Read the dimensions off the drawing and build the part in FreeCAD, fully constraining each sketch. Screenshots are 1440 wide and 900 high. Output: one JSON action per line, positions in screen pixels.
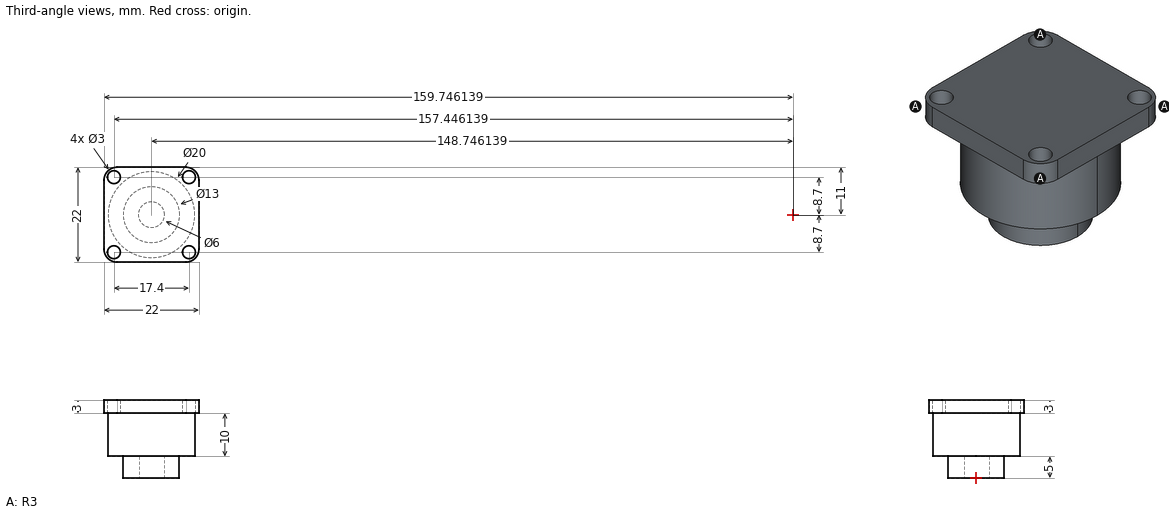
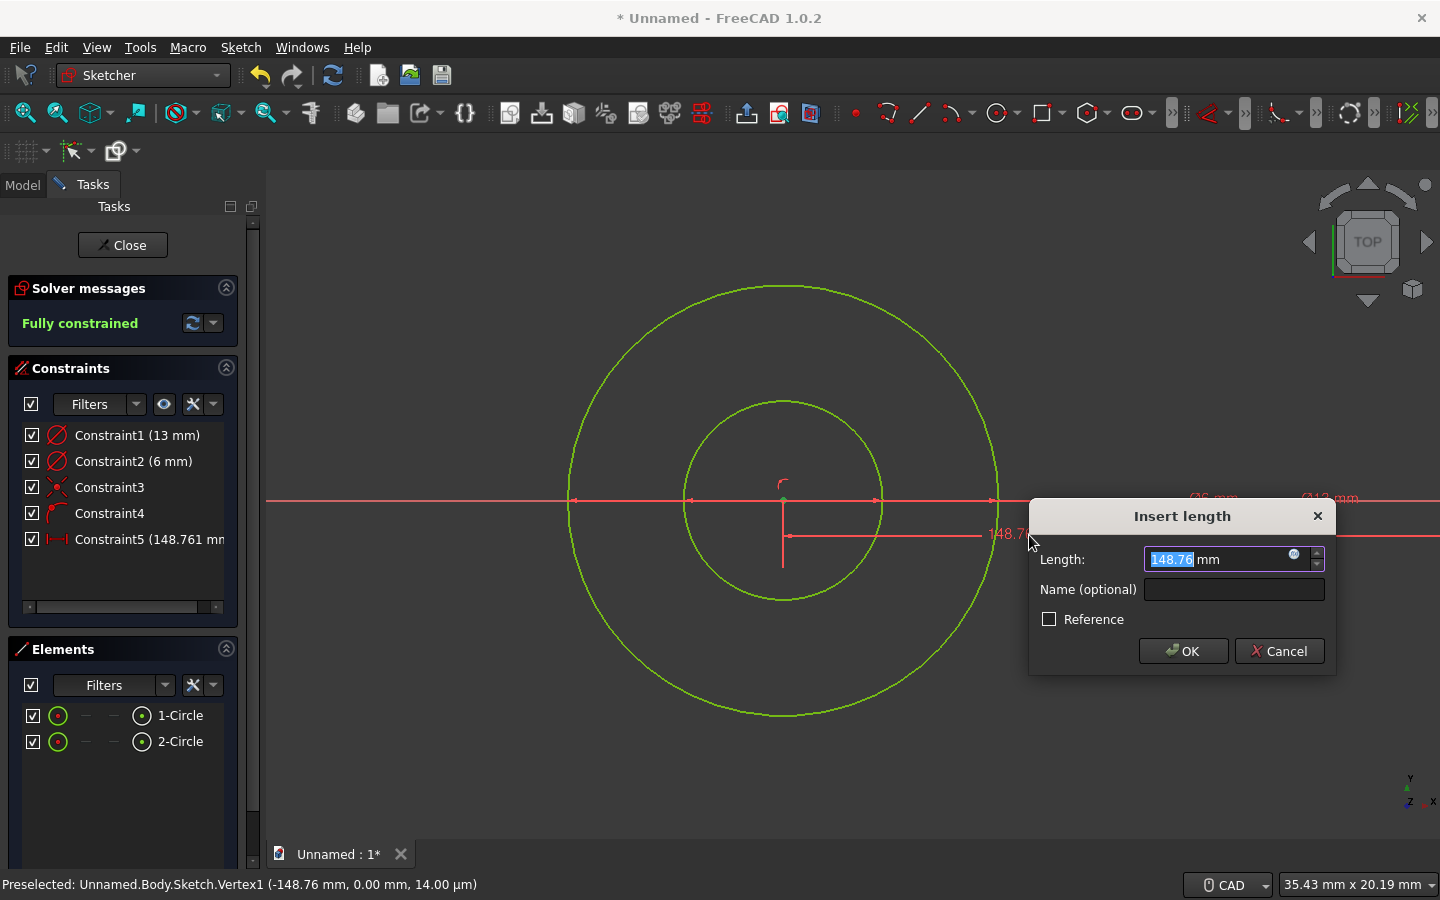
{"action": "type", "text": "148.746139"}
{"action": "key", "text": "Return"}
{"action": "key", "text": "Escape"}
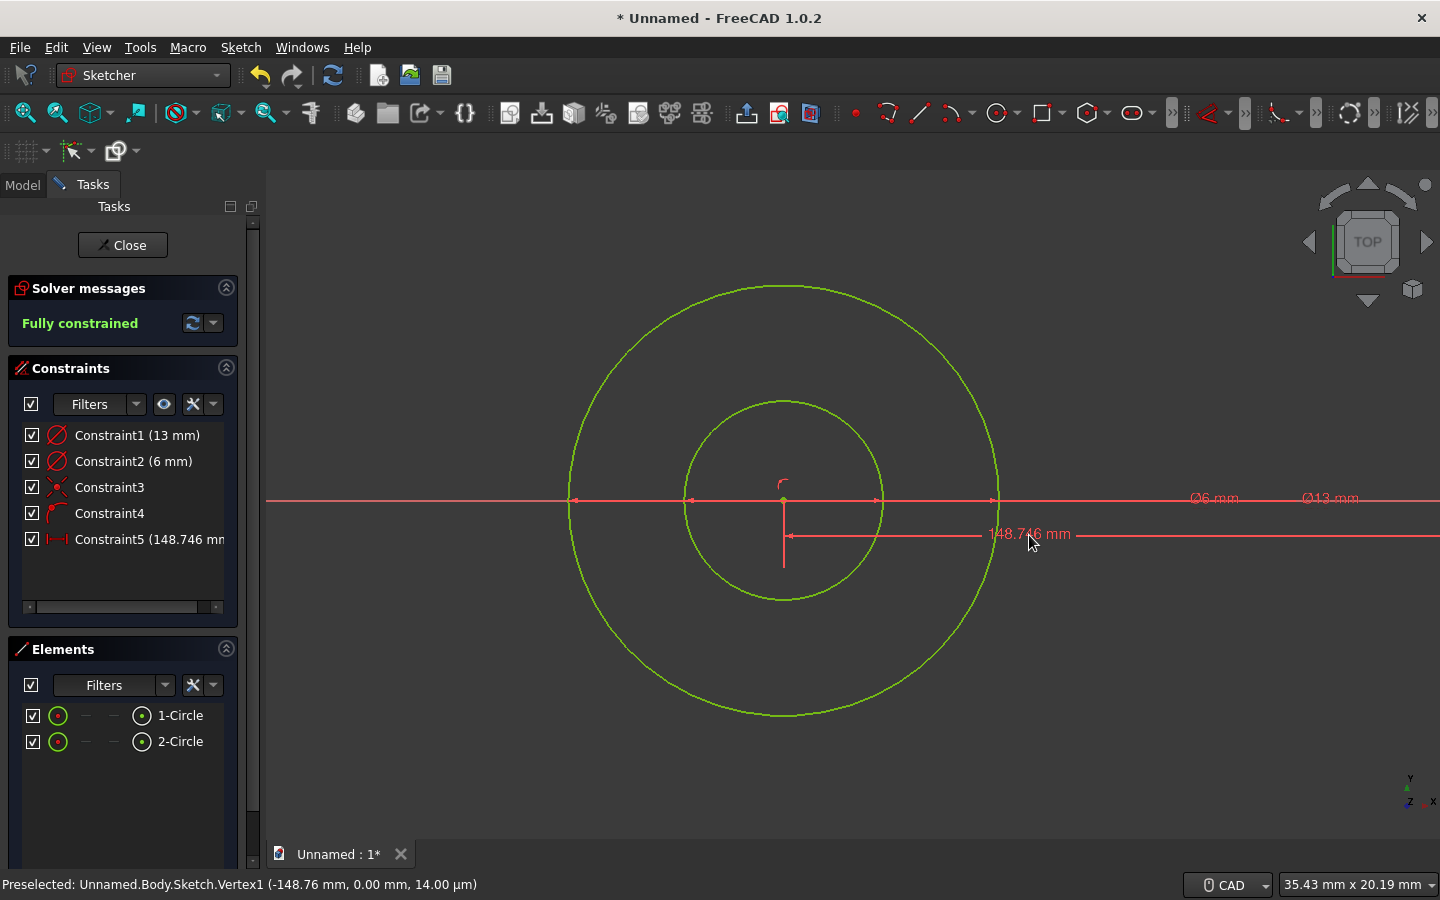
{"action": "left_click", "coordinate": [123, 245]}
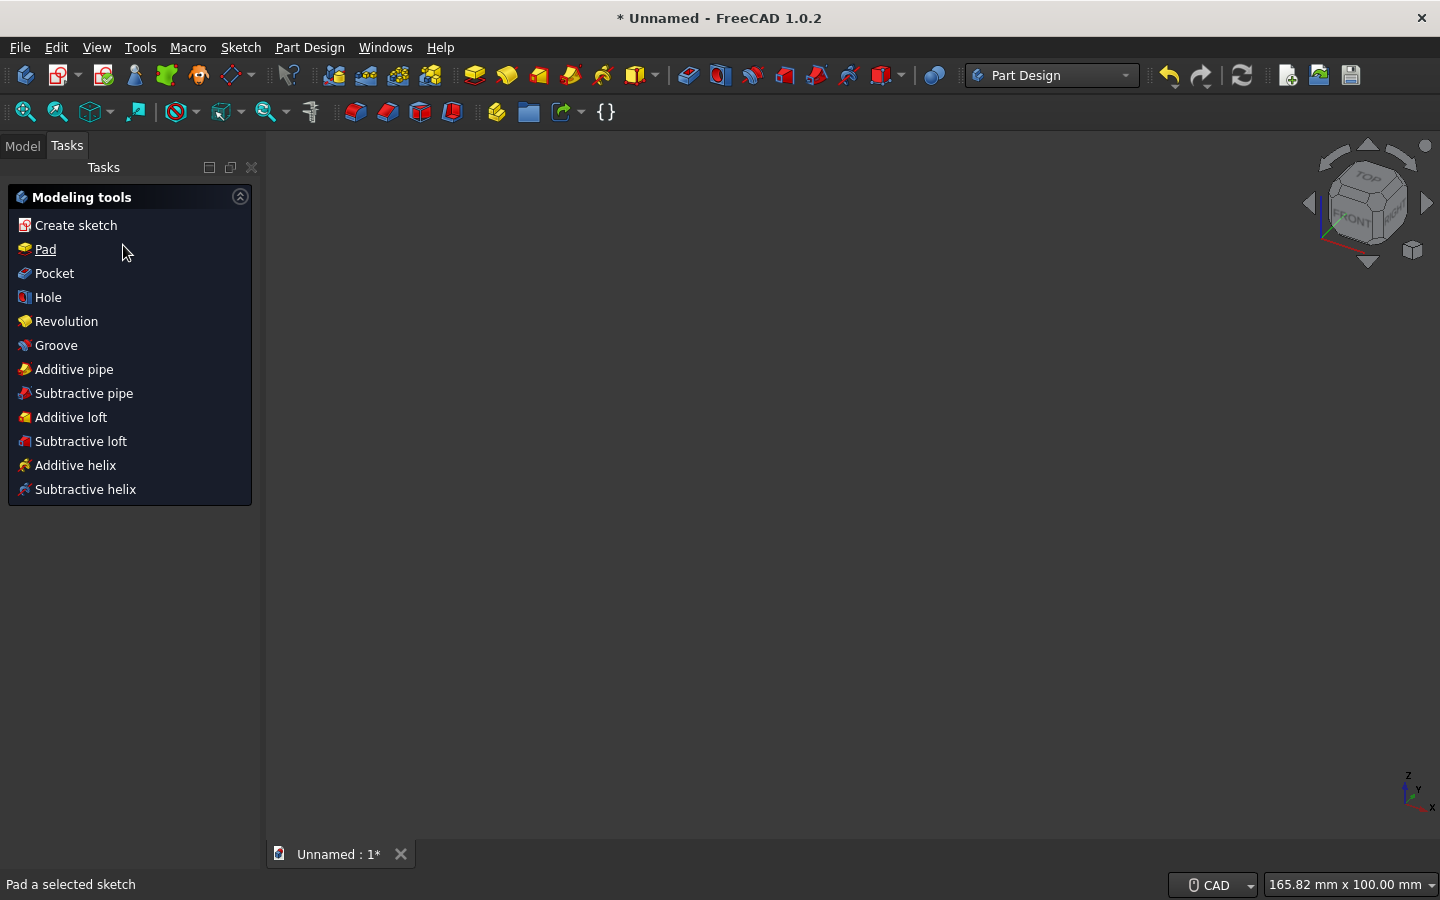
{"action": "left_click", "coordinate": [476, 76]}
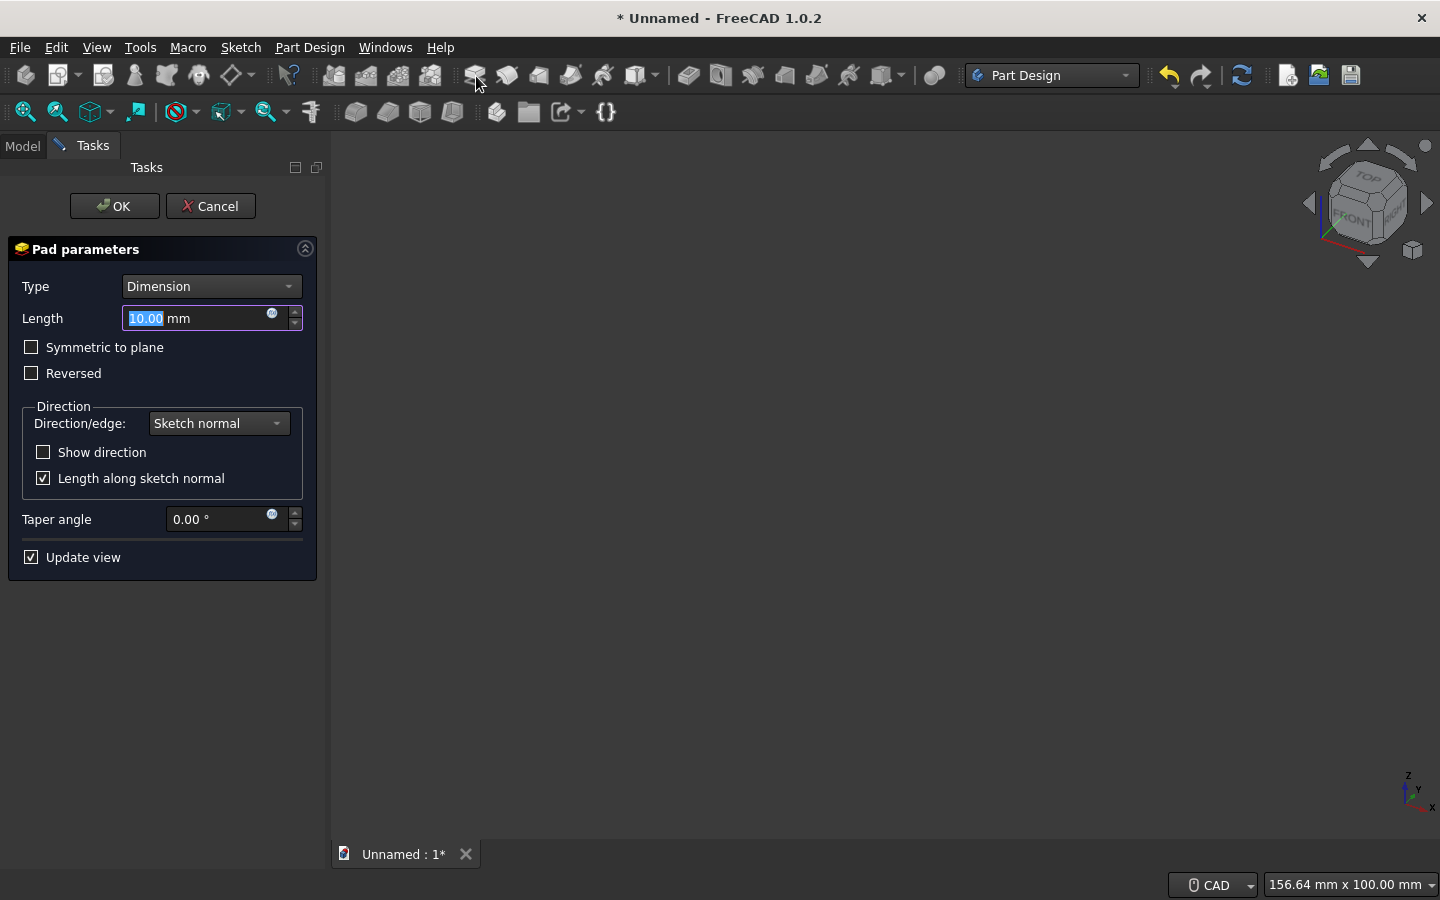
{"action": "type", "text": "5"}
{"action": "key", "text": "Tab"}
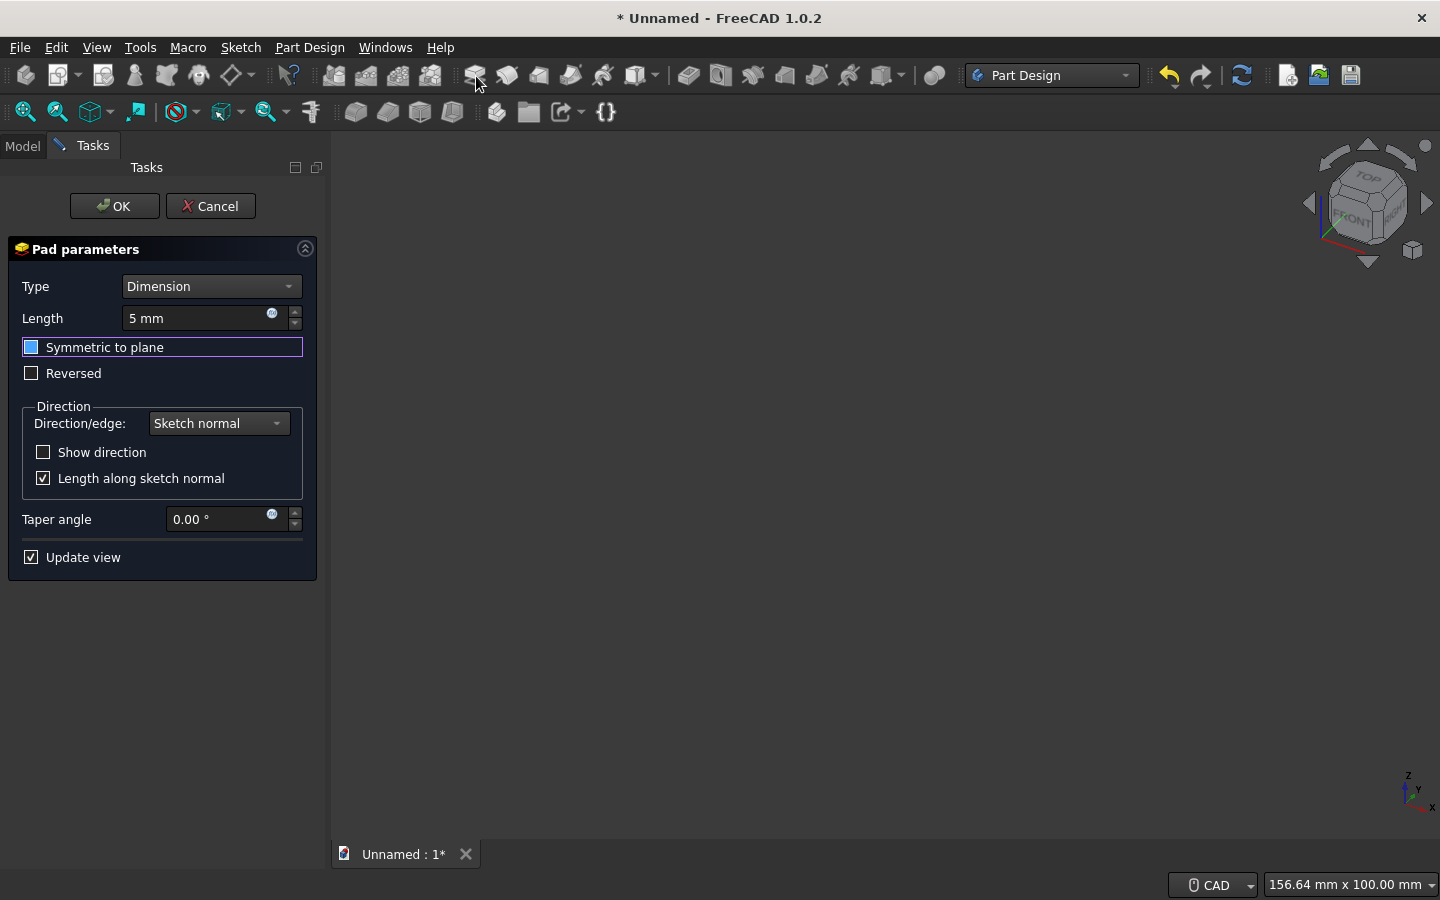
{"action": "left_click", "coordinate": [115, 206]}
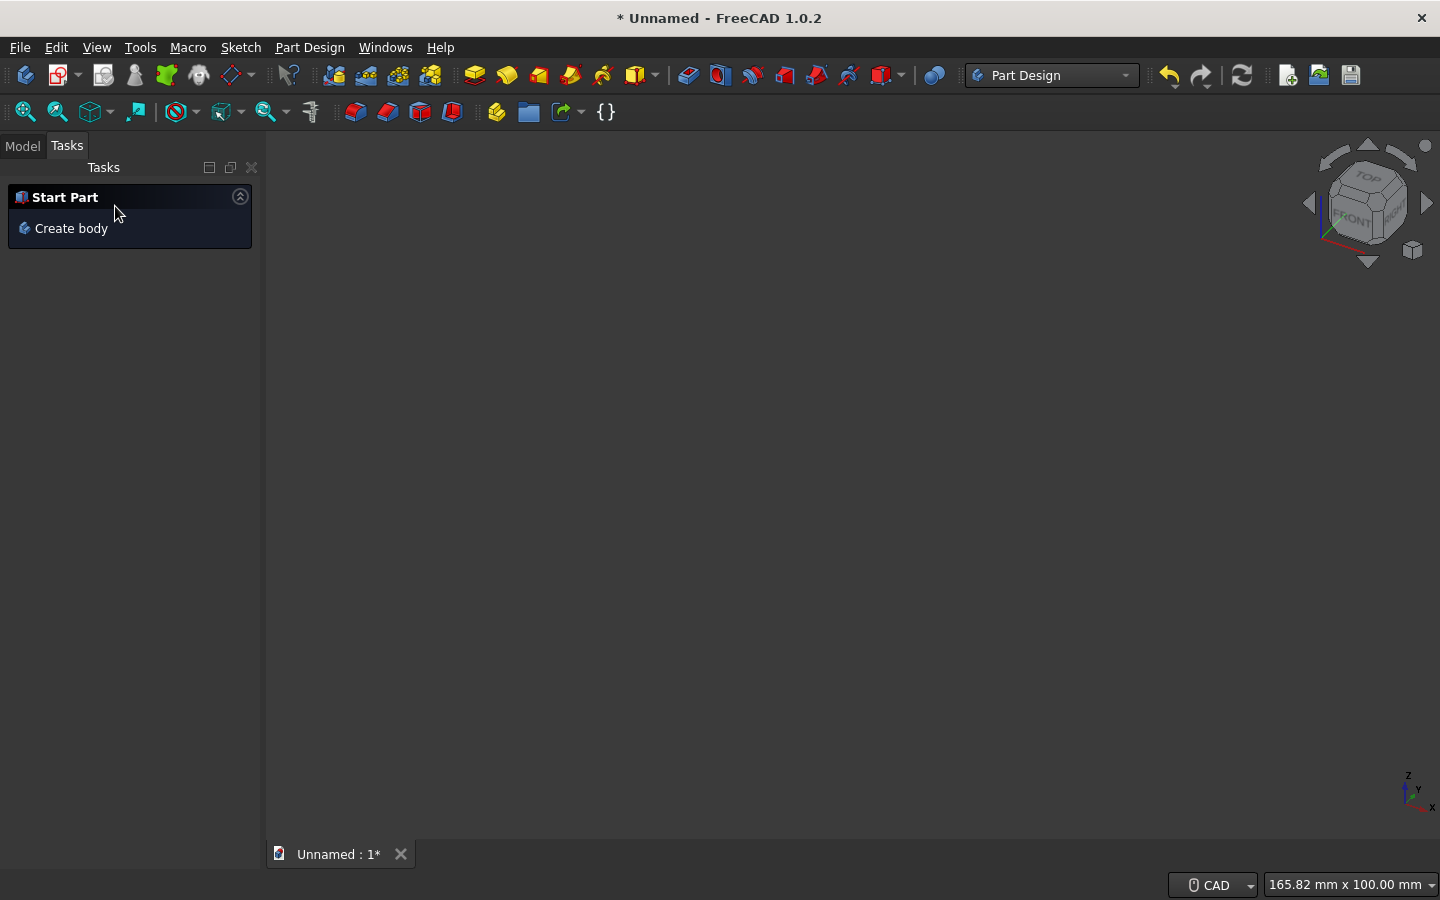
{"action": "left_click", "coordinate": [26, 112]}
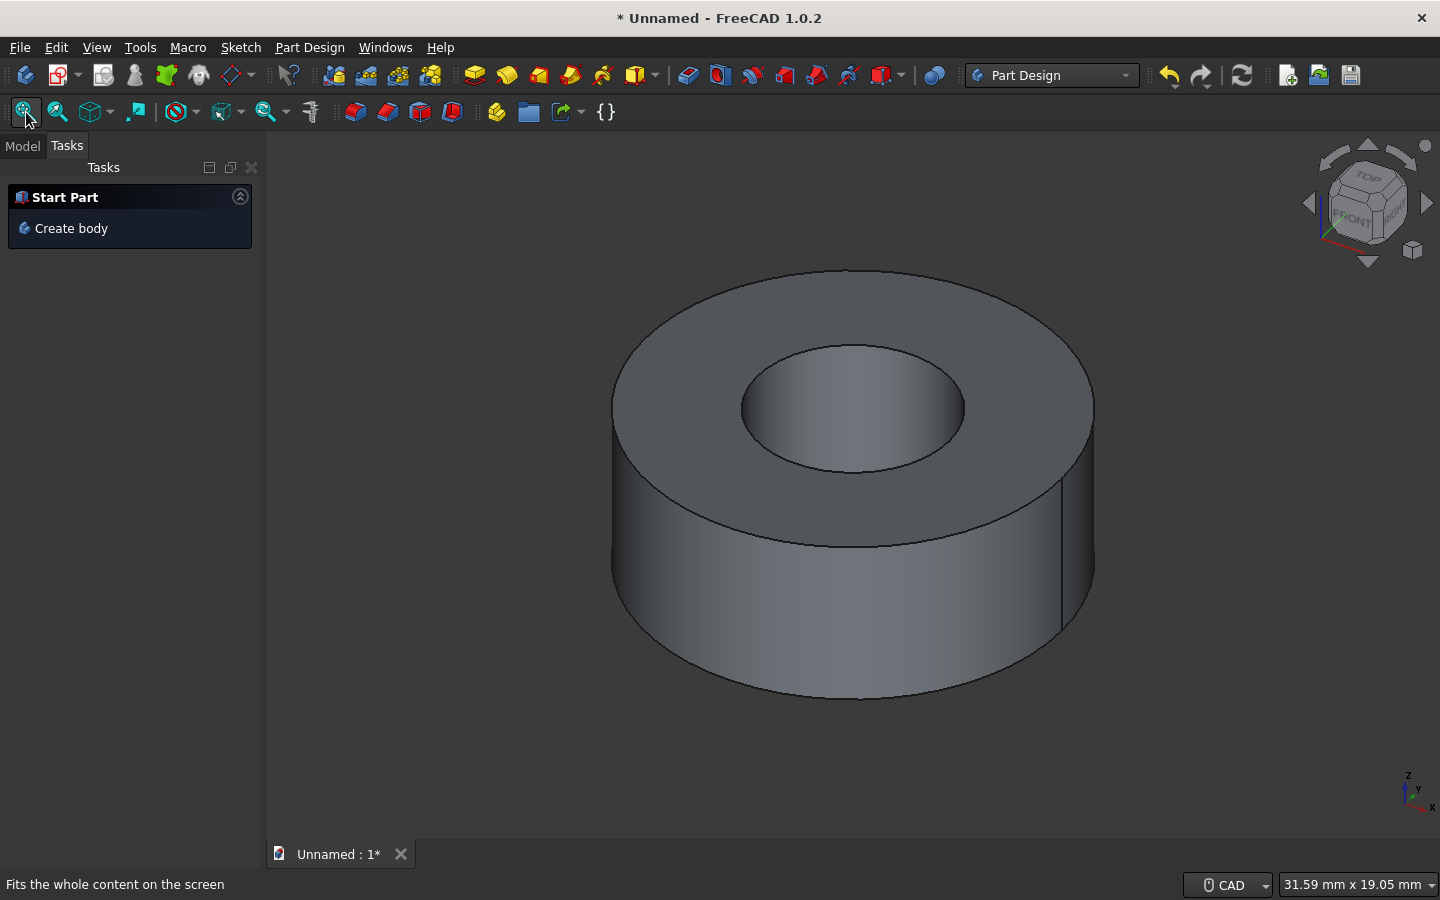
{"action": "left_click", "coordinate": [904, 516]}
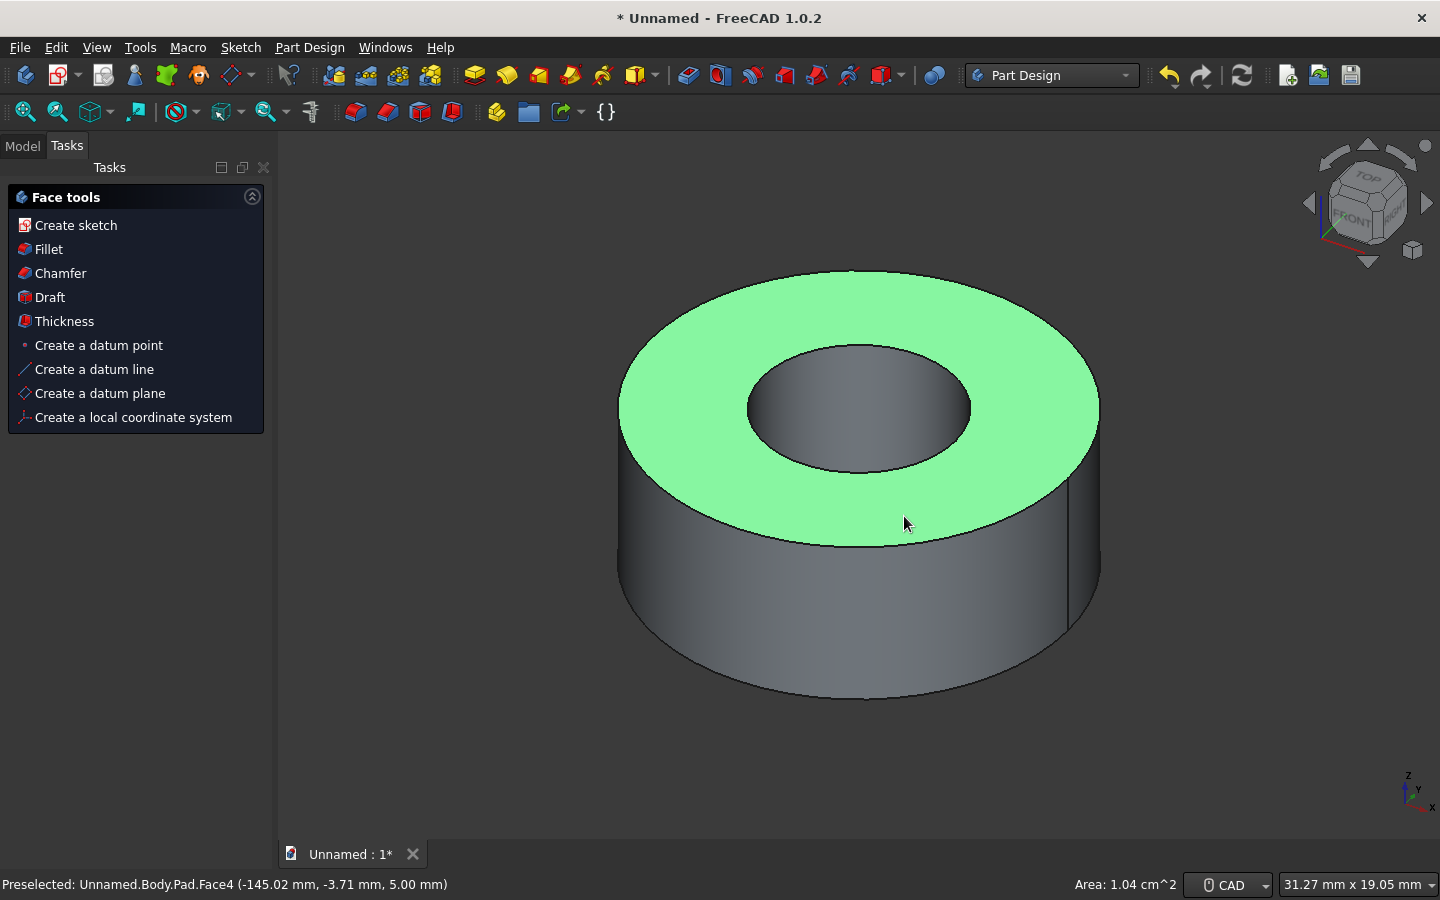
{"action": "left_click", "coordinate": [58, 76]}